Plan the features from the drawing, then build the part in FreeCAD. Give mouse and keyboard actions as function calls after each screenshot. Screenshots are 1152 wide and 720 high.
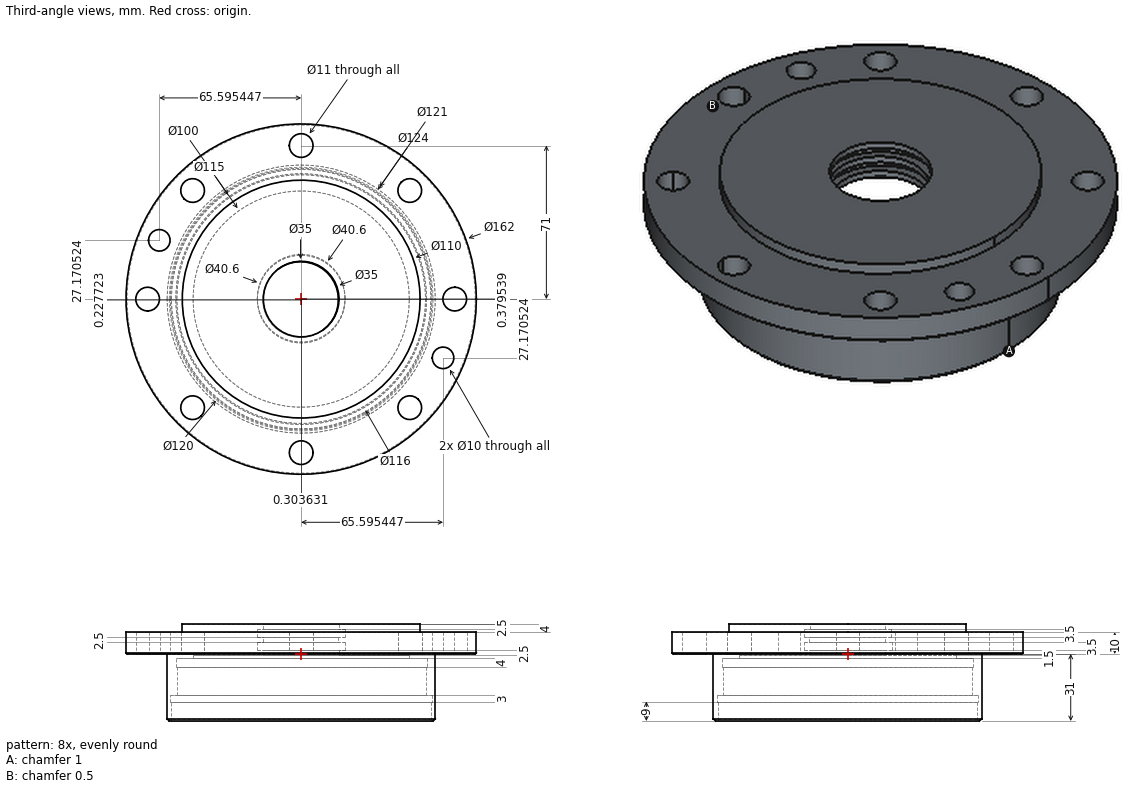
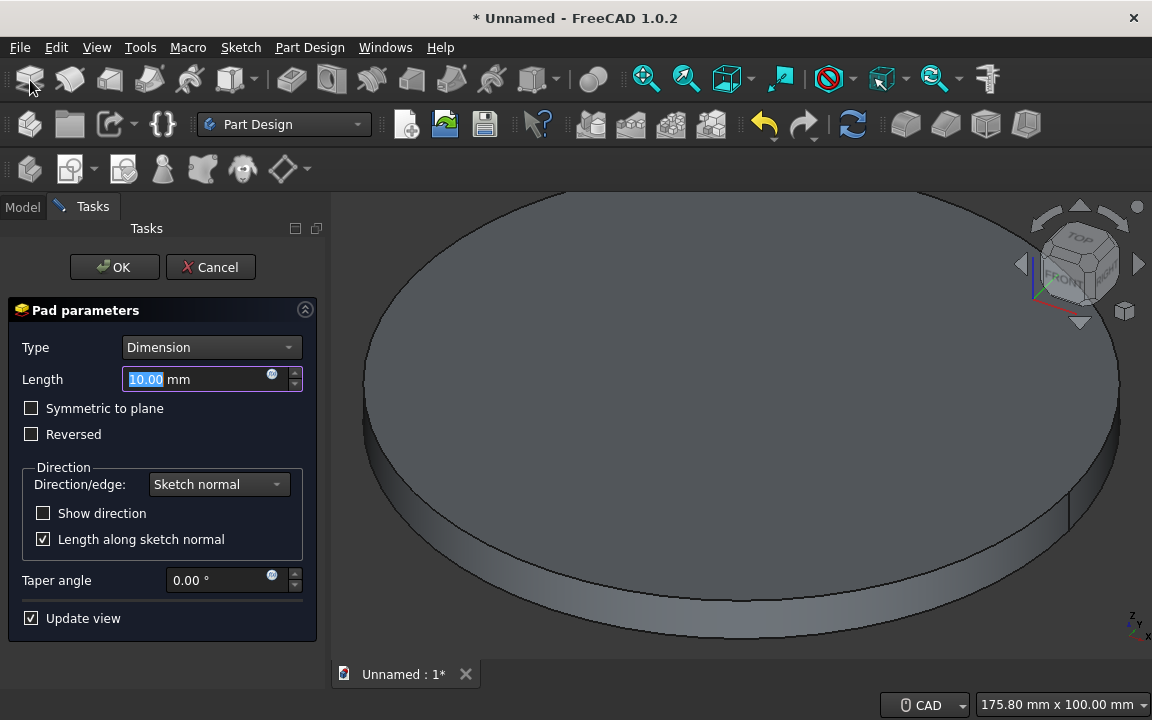
text(10)
key(Tab)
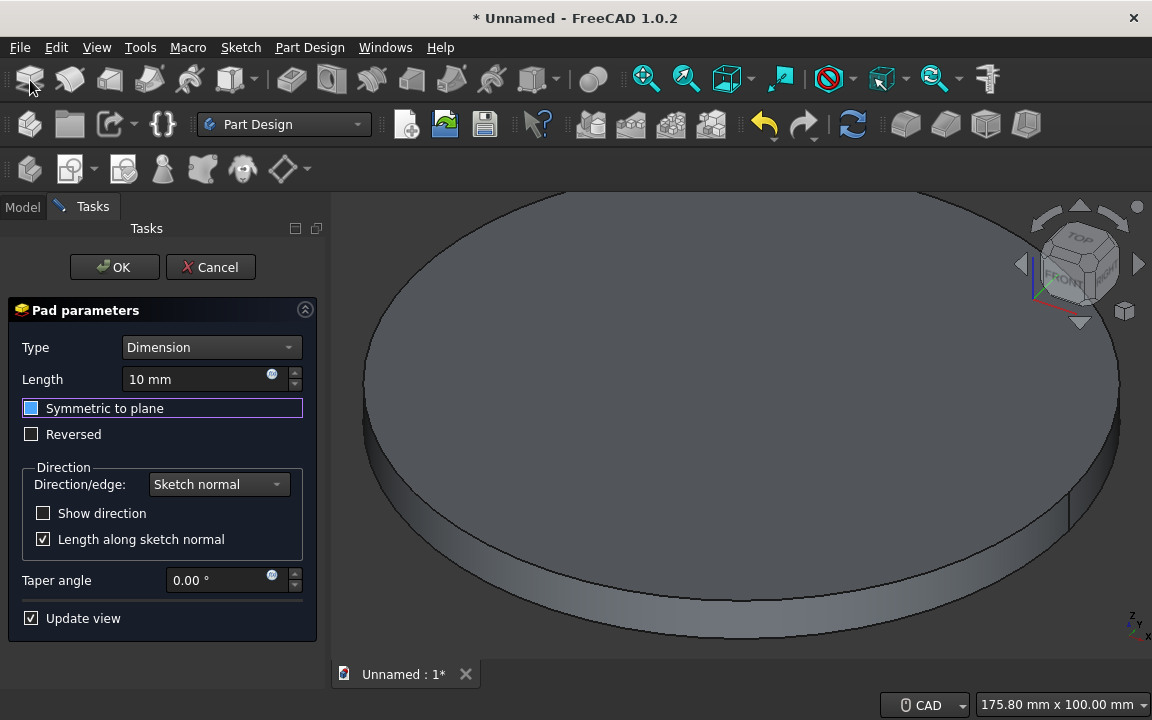
click(115, 267)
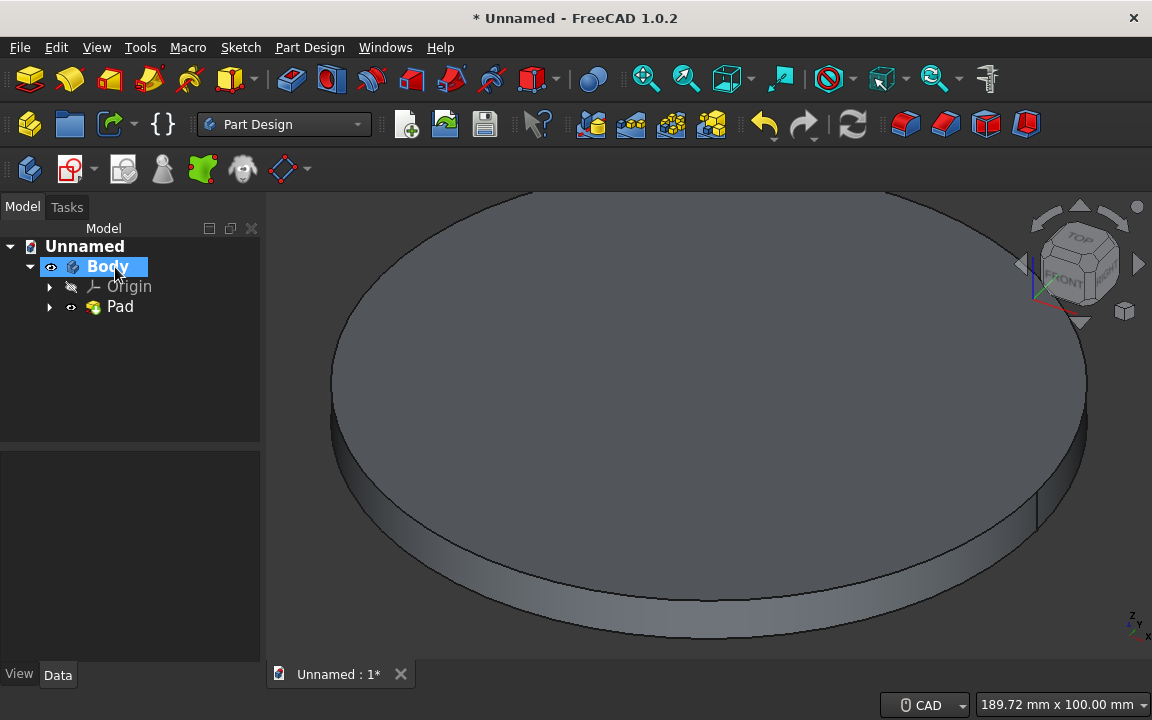
click(648, 80)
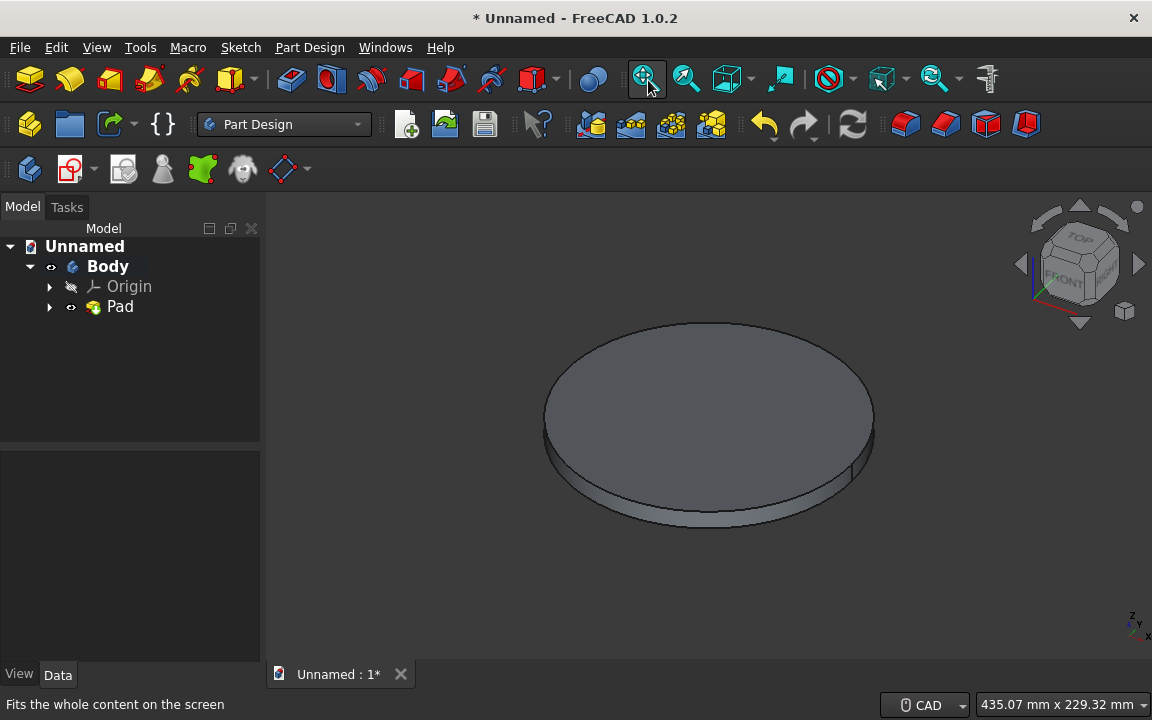
click(709, 416)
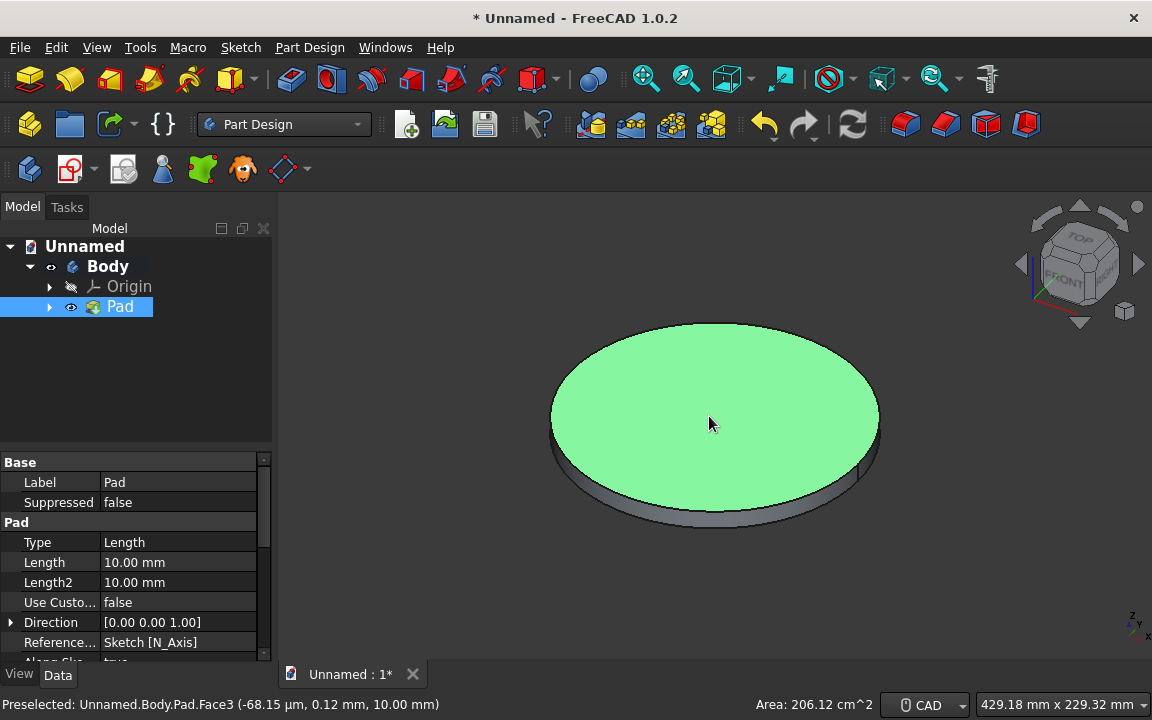
click(70, 170)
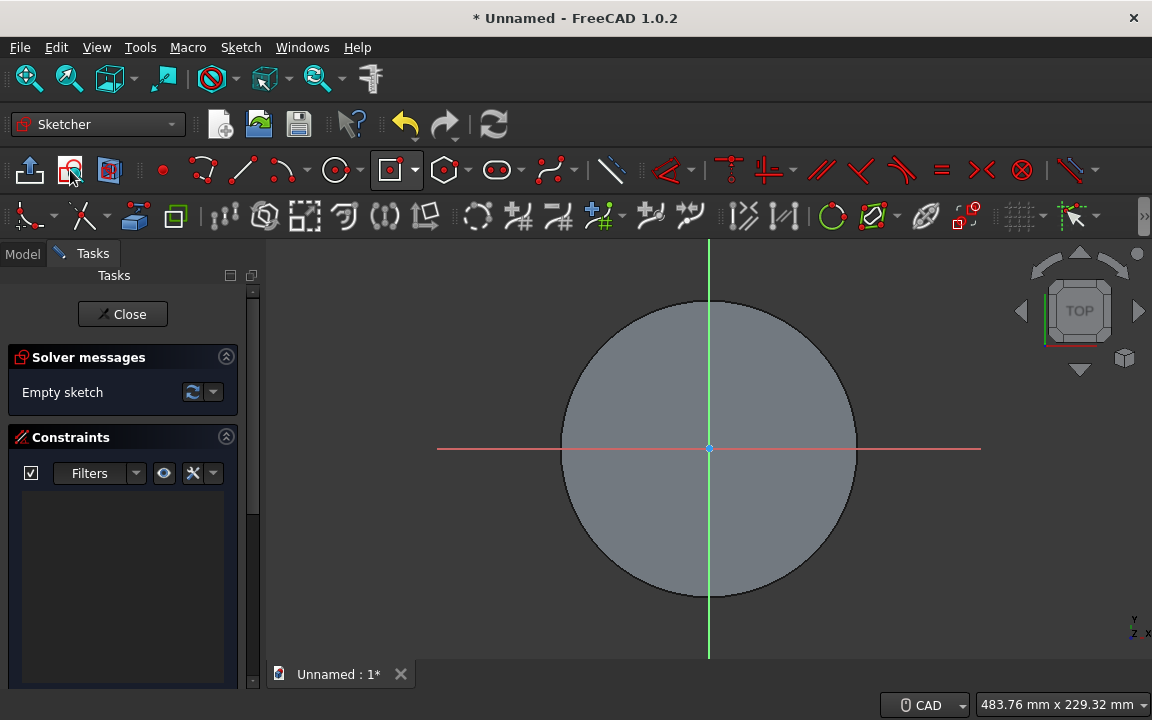
click(336, 170)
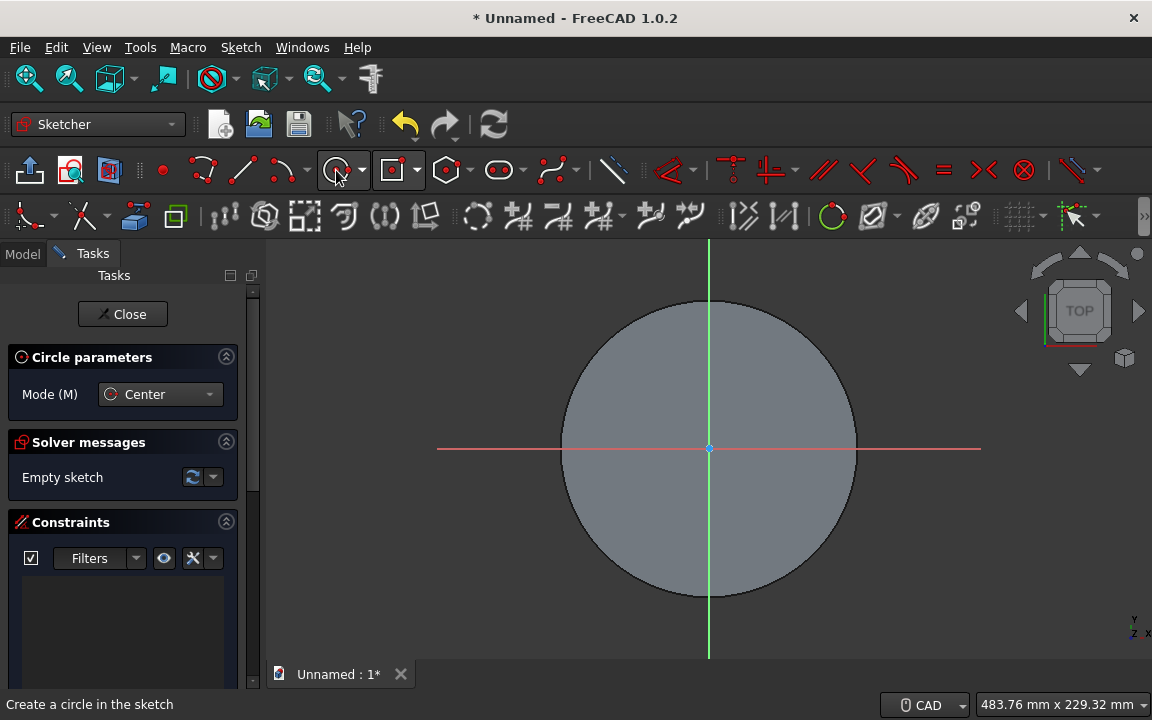
click(709, 449)
click(780, 378)
key(Escape)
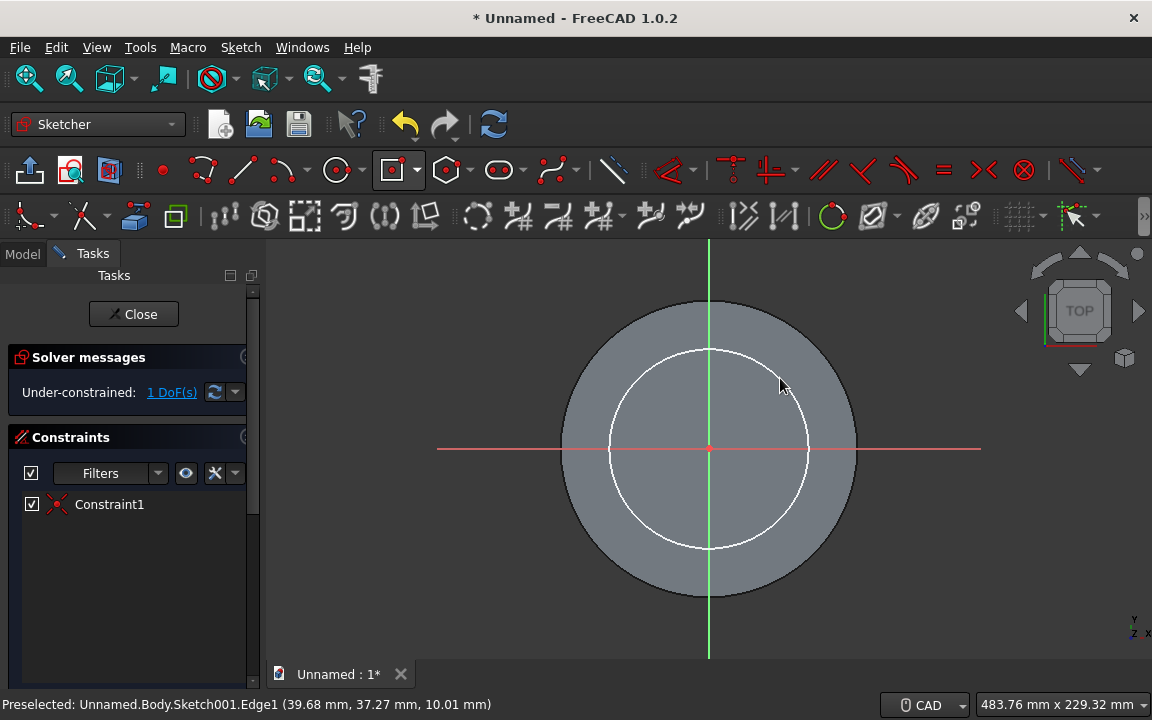
click(668, 170)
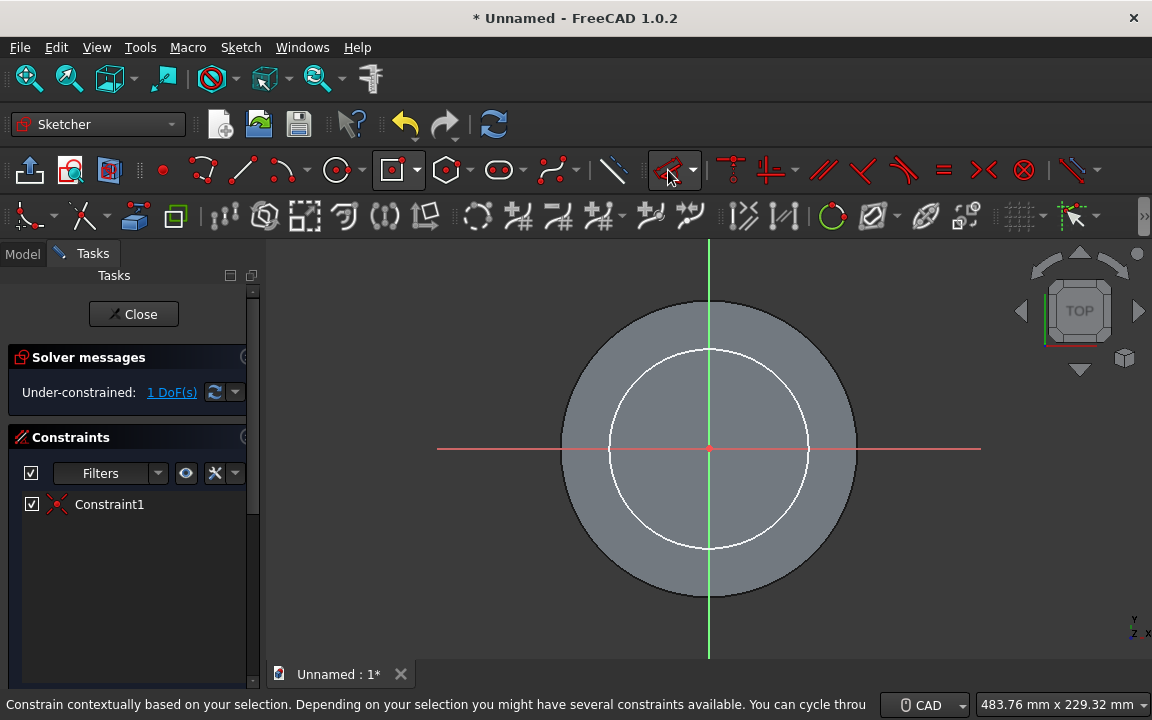
click(779, 378)
click(801, 355)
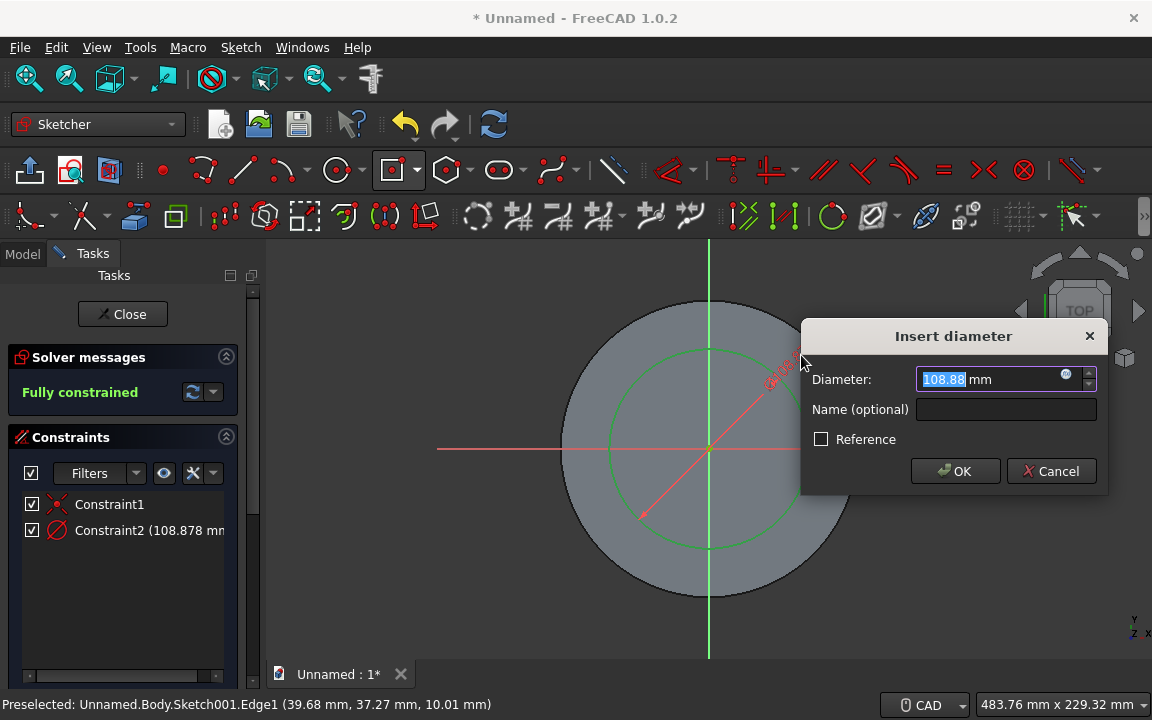
text(110)
key(Return)
key(Escape)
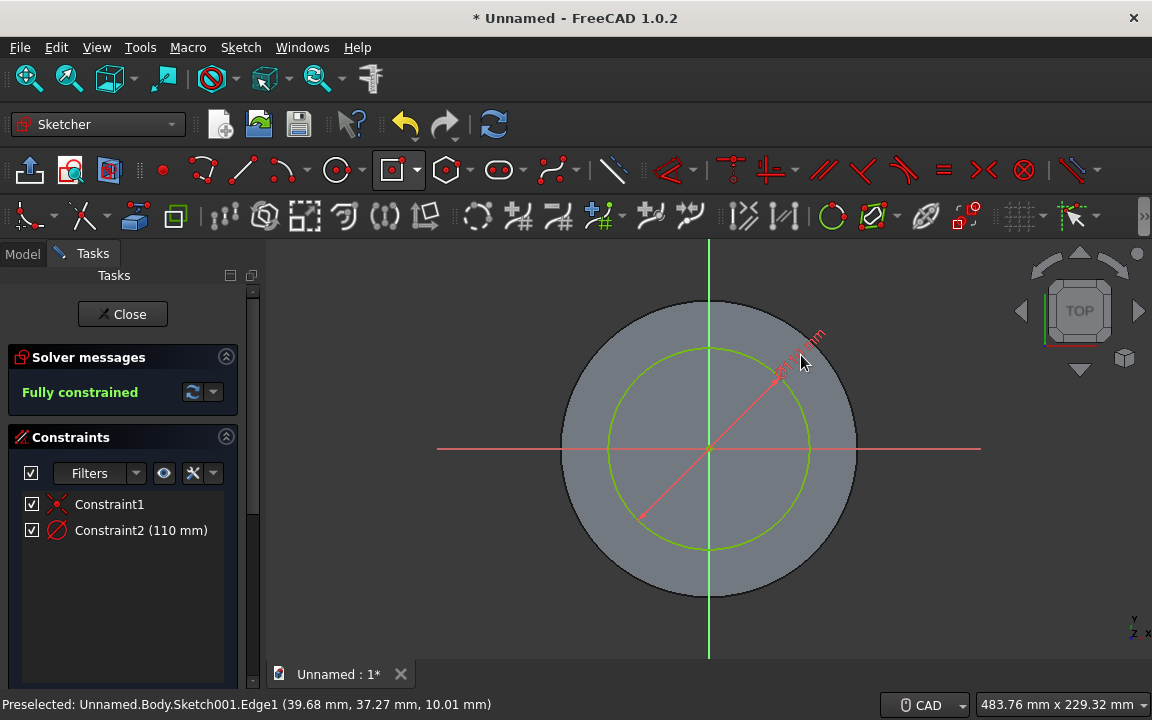
click(123, 314)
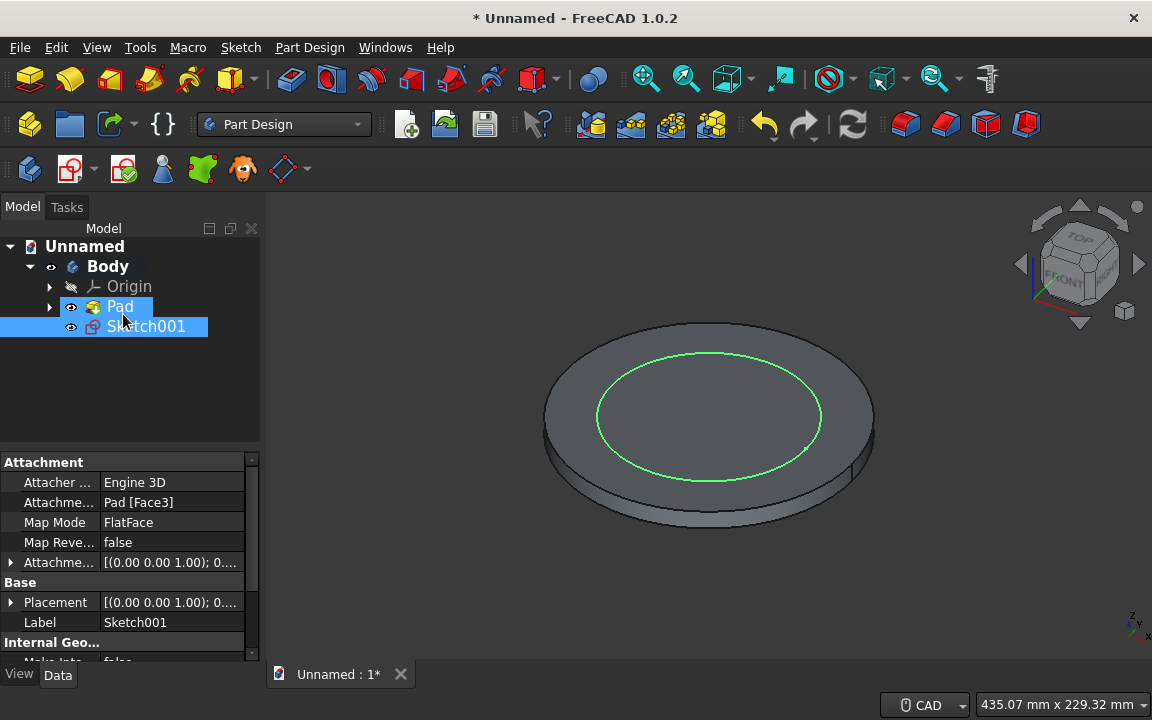
click(30, 80)